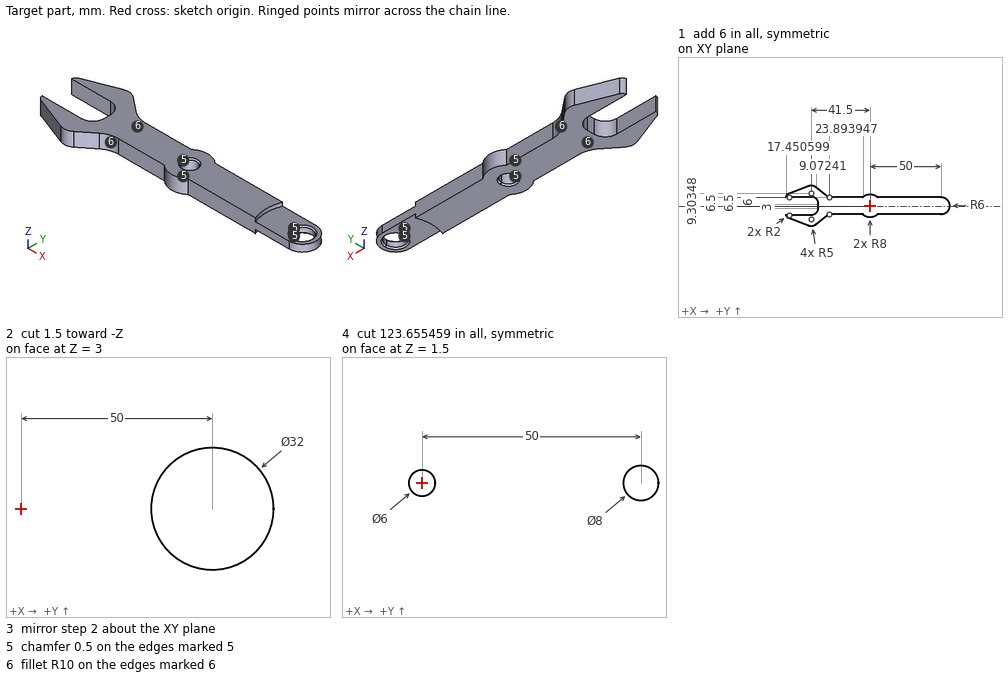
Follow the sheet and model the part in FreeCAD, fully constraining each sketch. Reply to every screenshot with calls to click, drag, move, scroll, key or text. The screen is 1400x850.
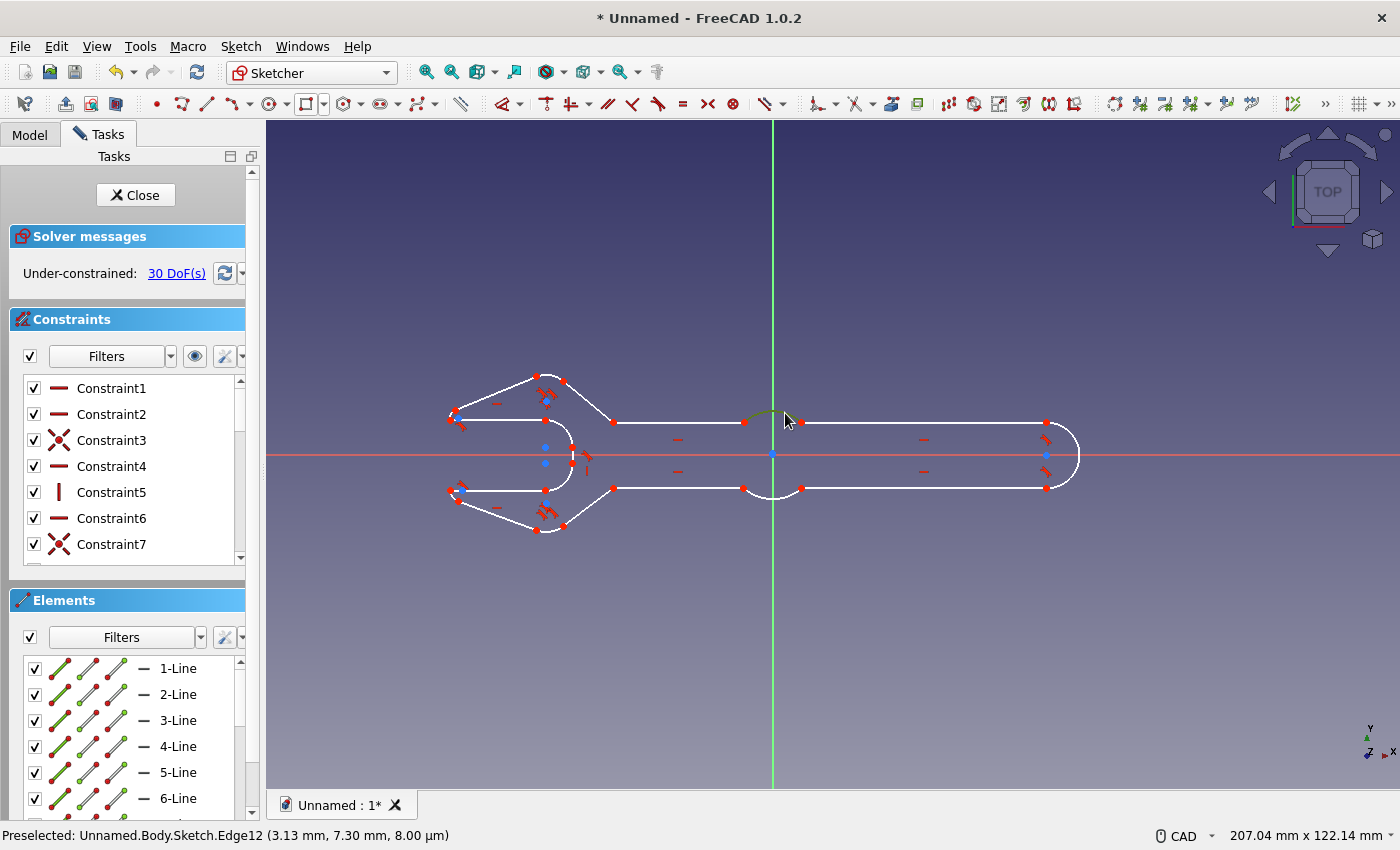
click(760, 497)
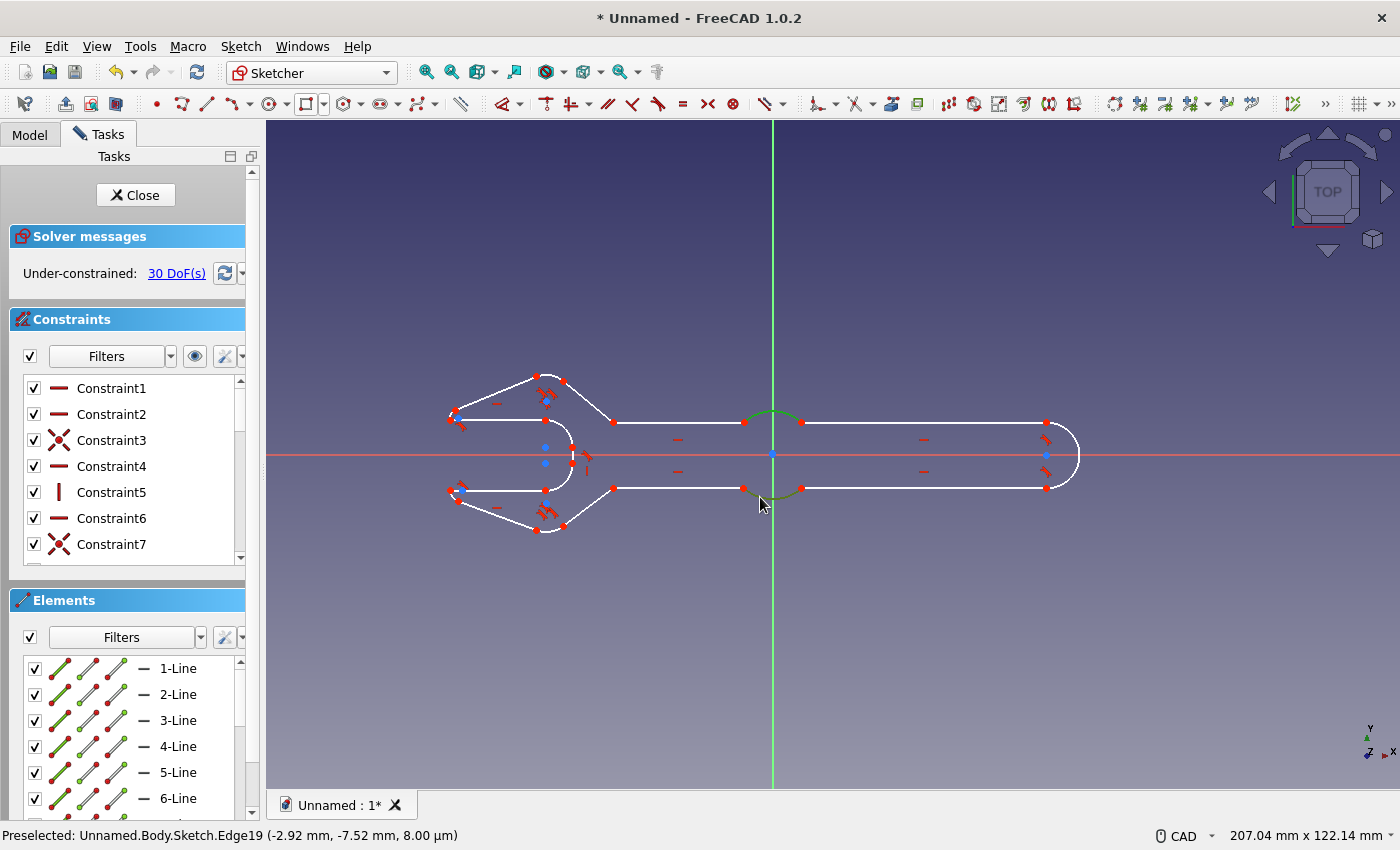
click(546, 104)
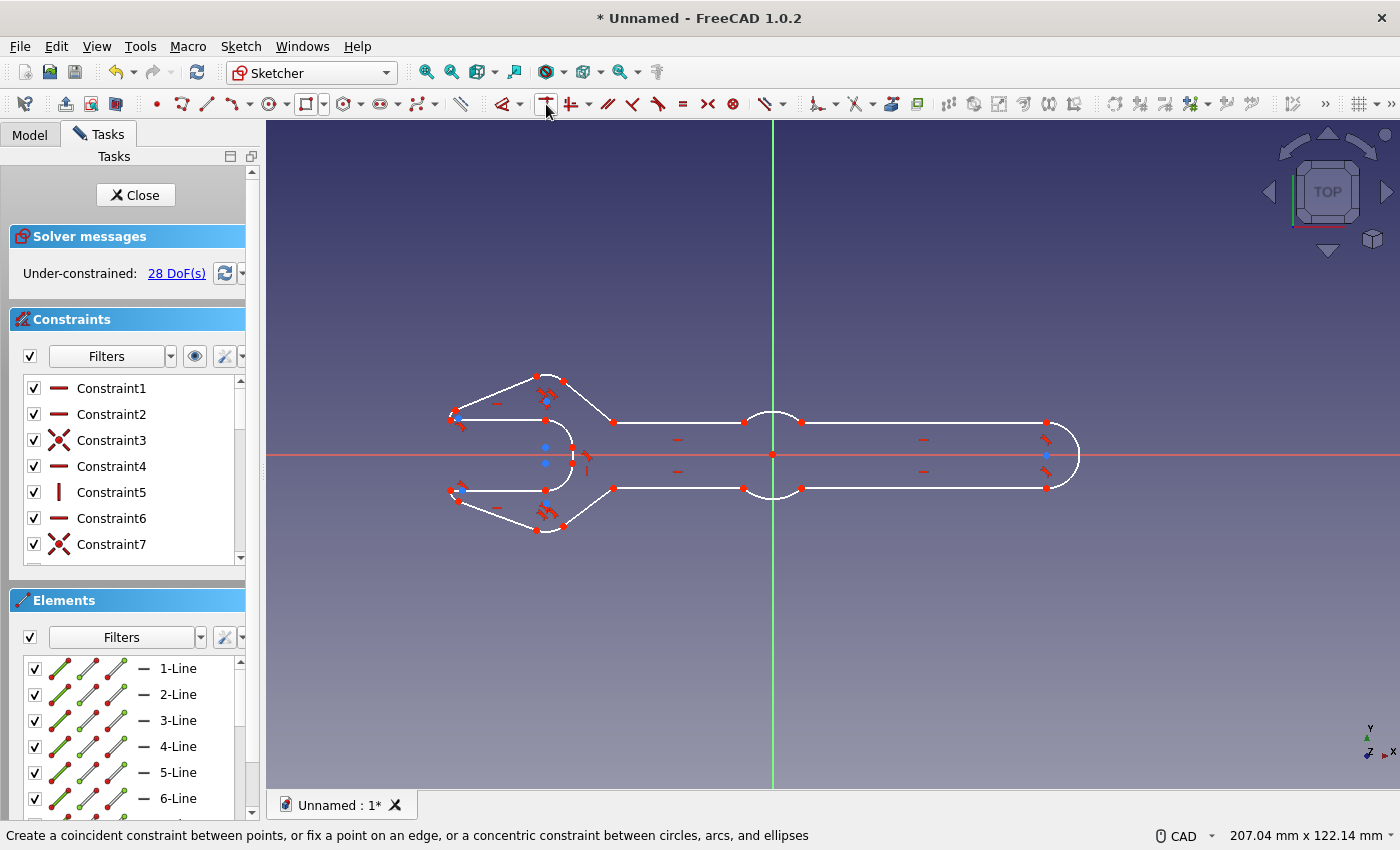
scroll(773, 455, up, 8)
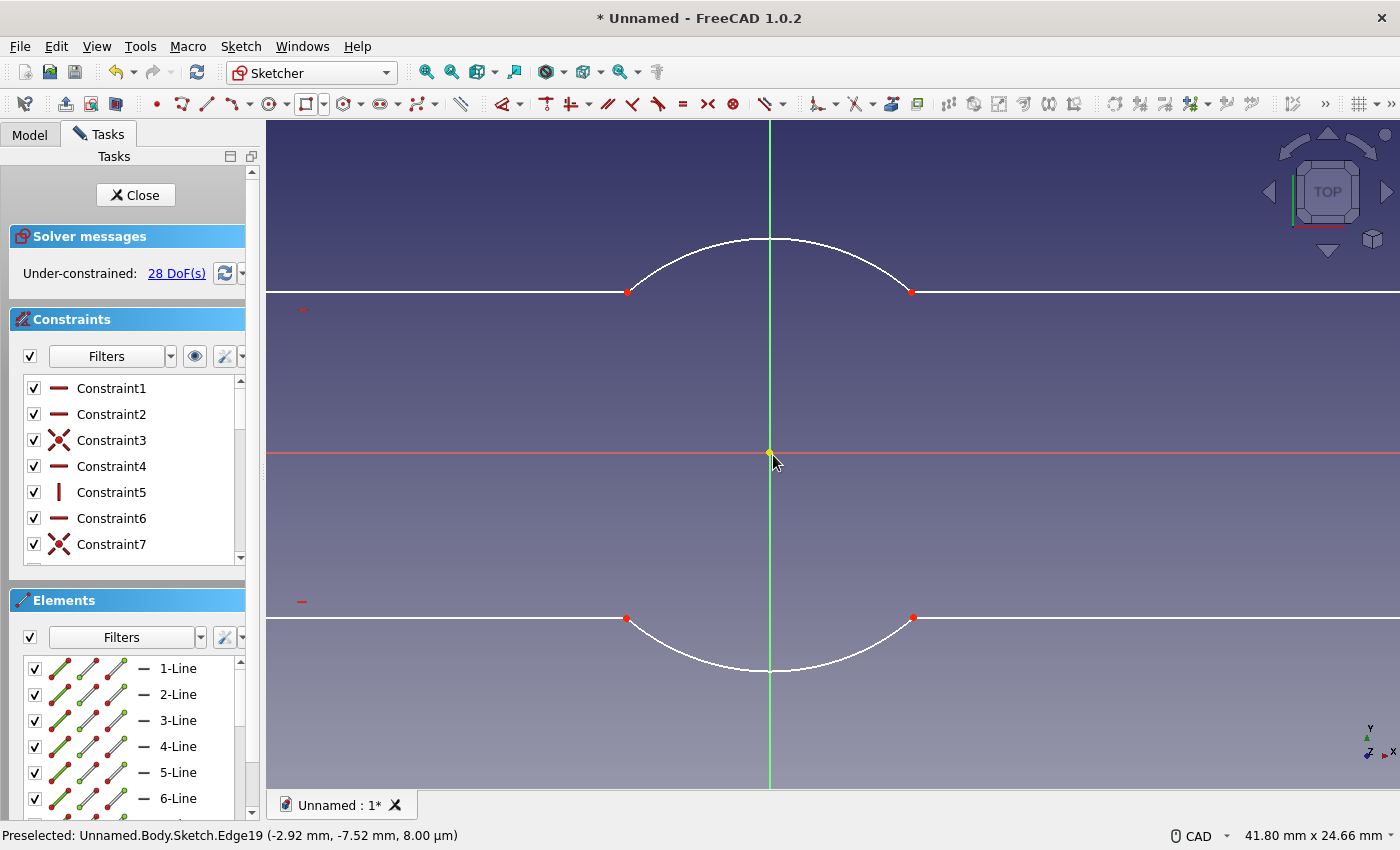
drag(760, 442, 780, 463)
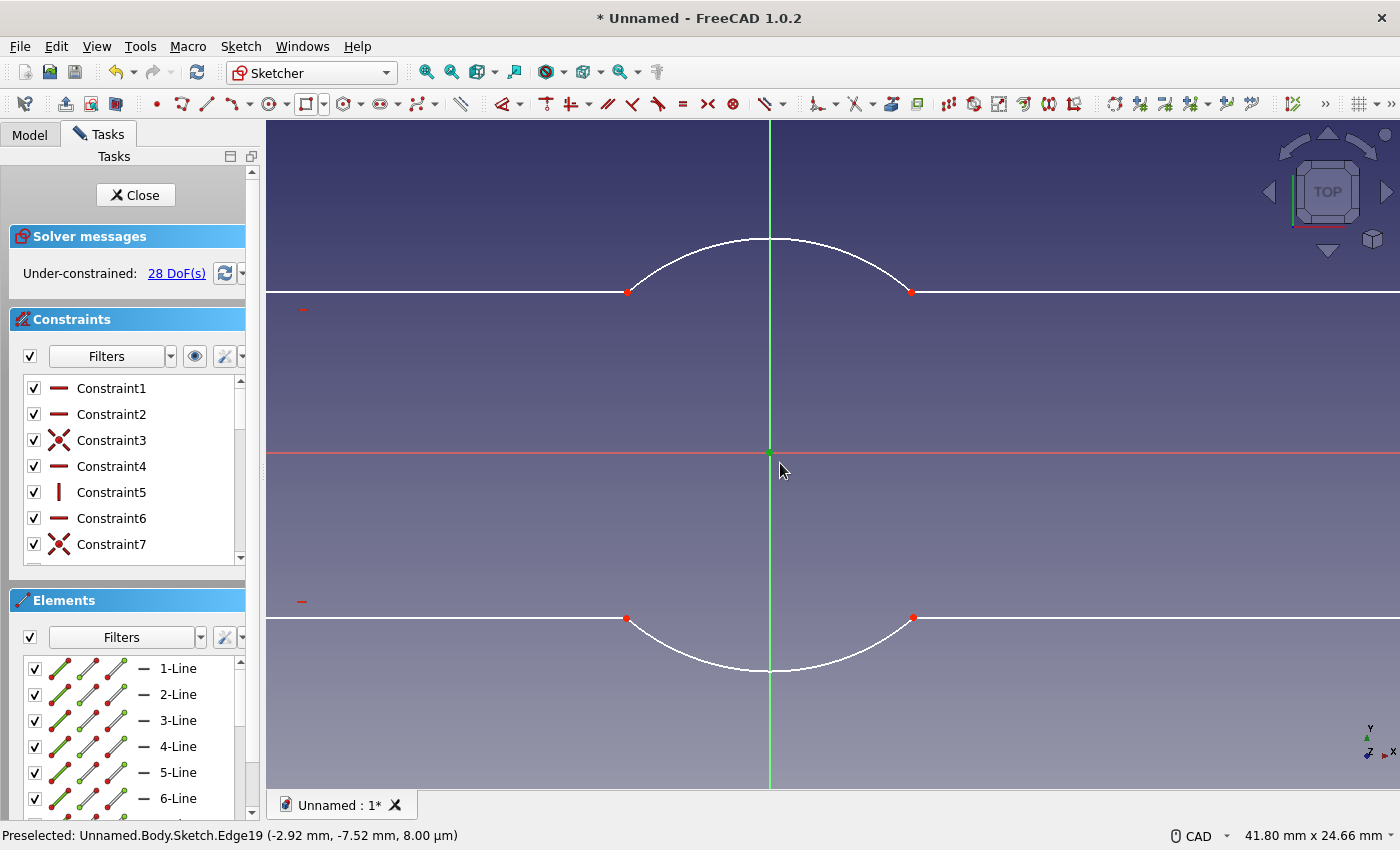
click(546, 104)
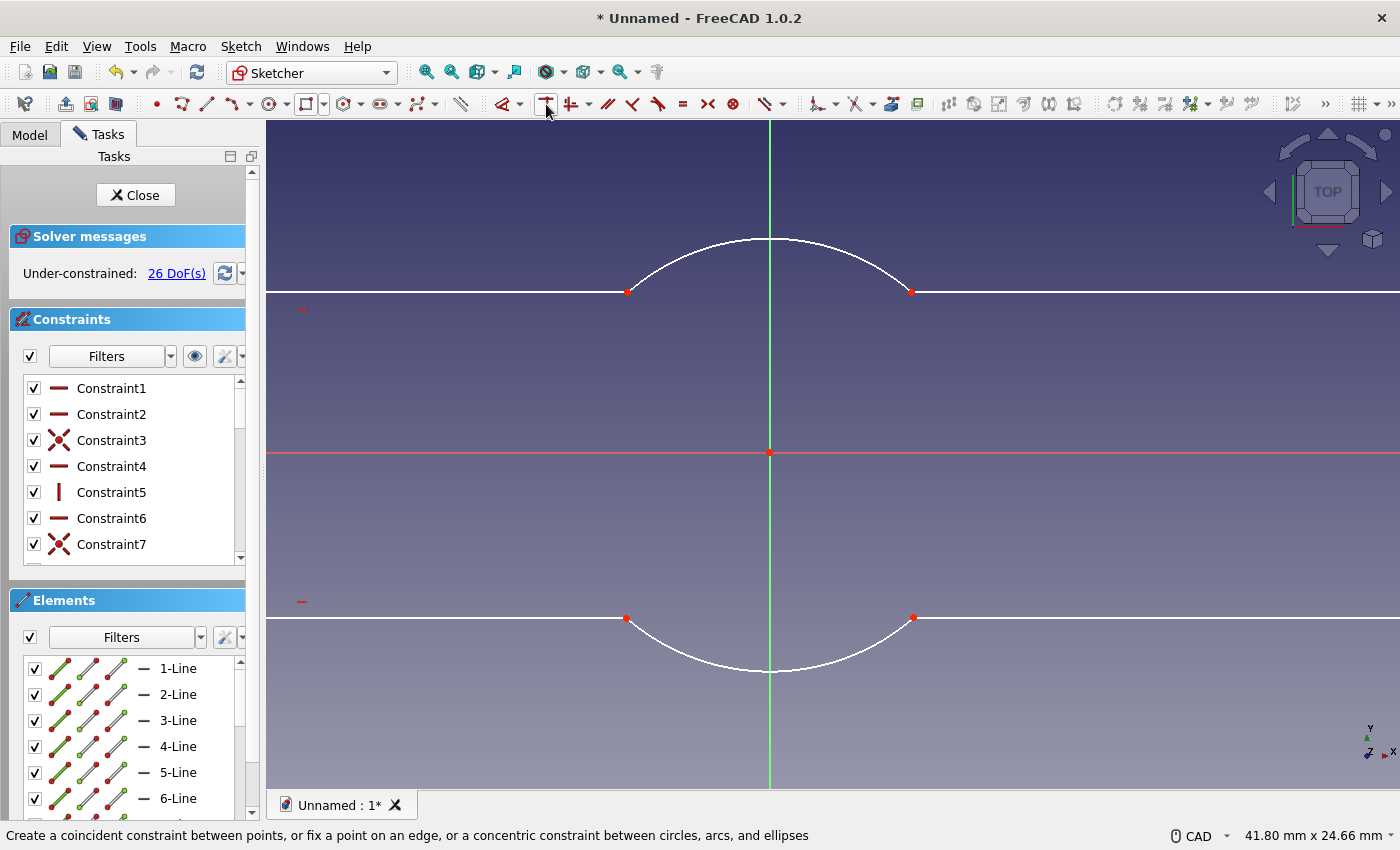
scroll(773, 455, down, 8)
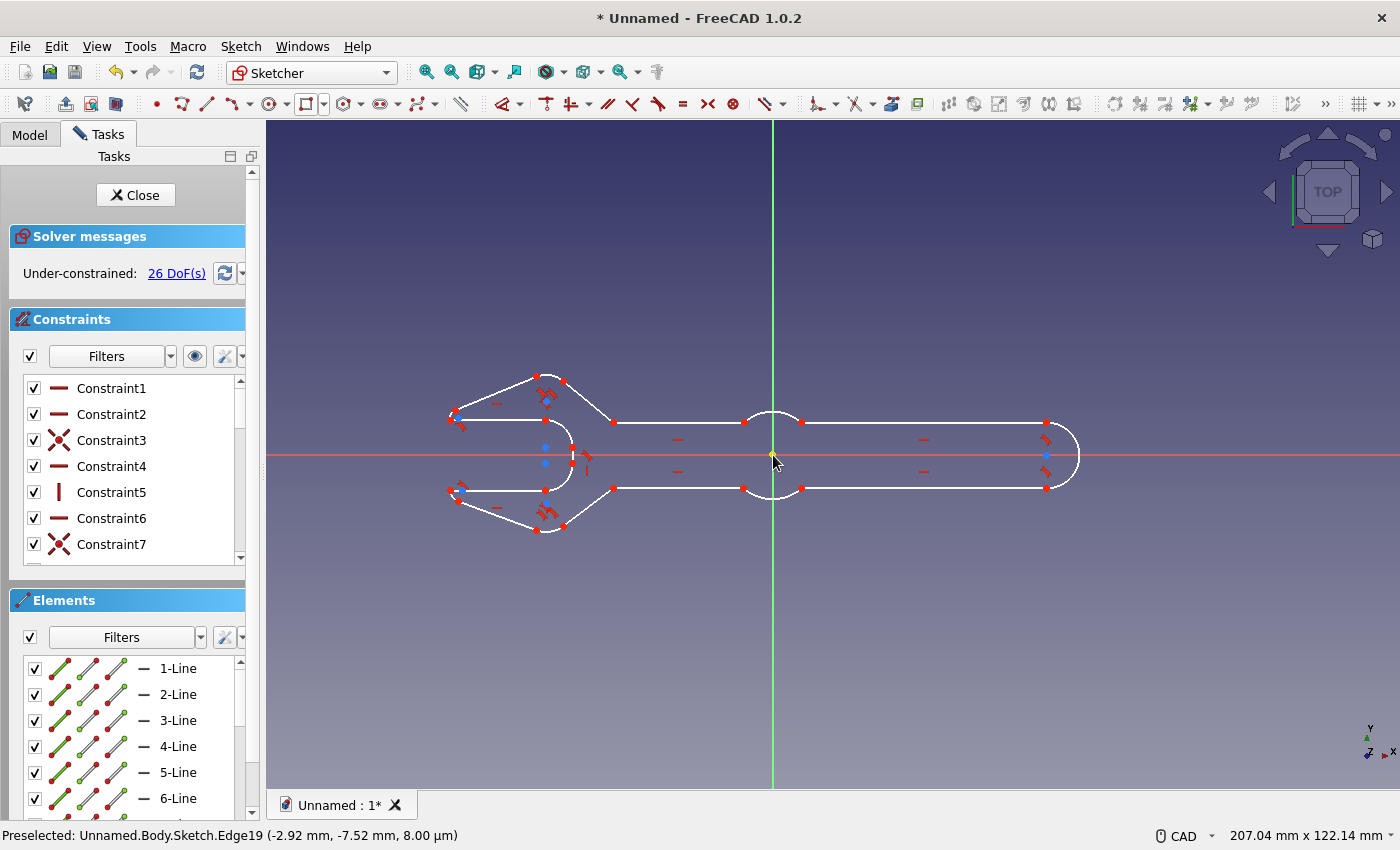
scroll(556, 377, up, 3)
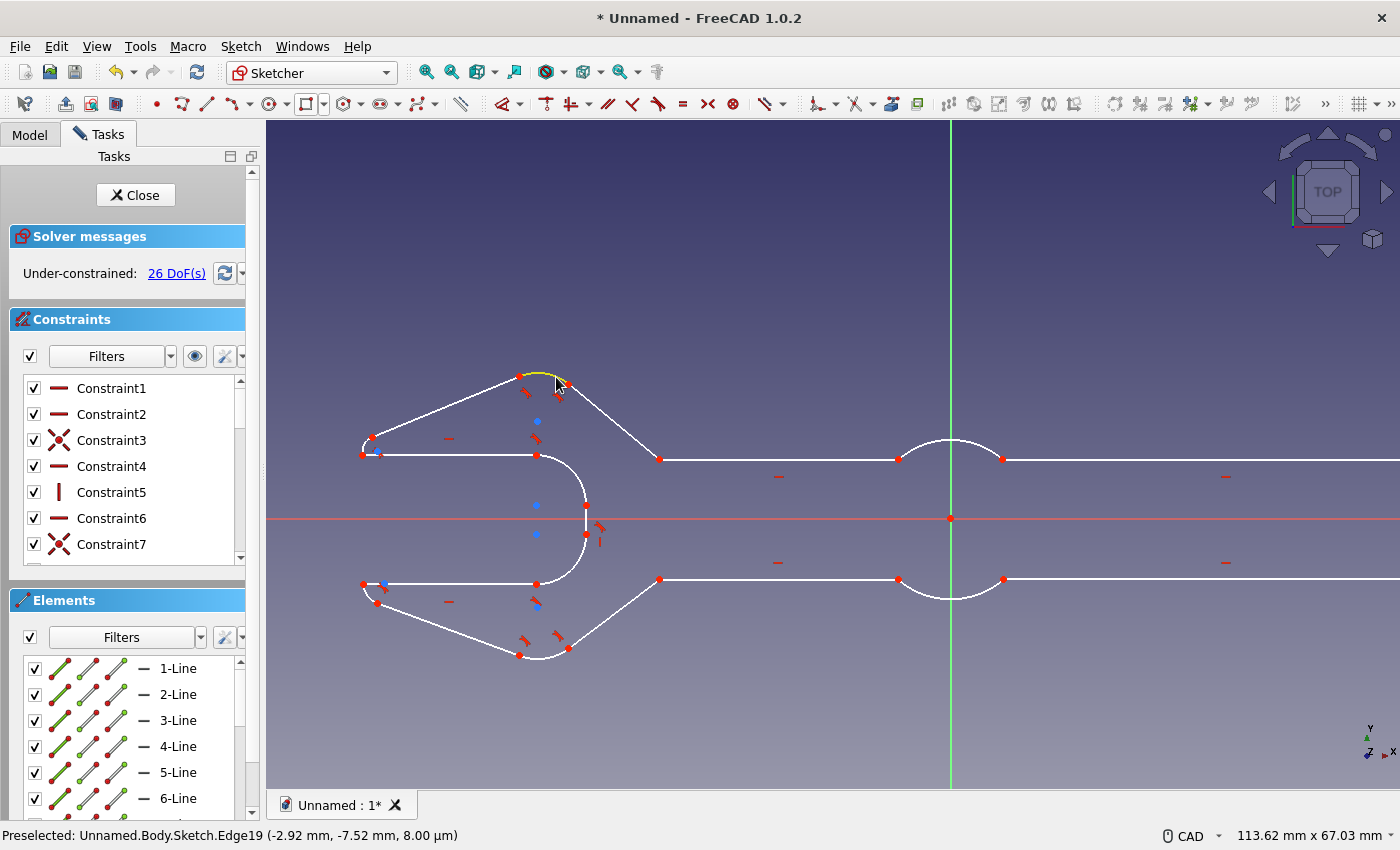
click(555, 376)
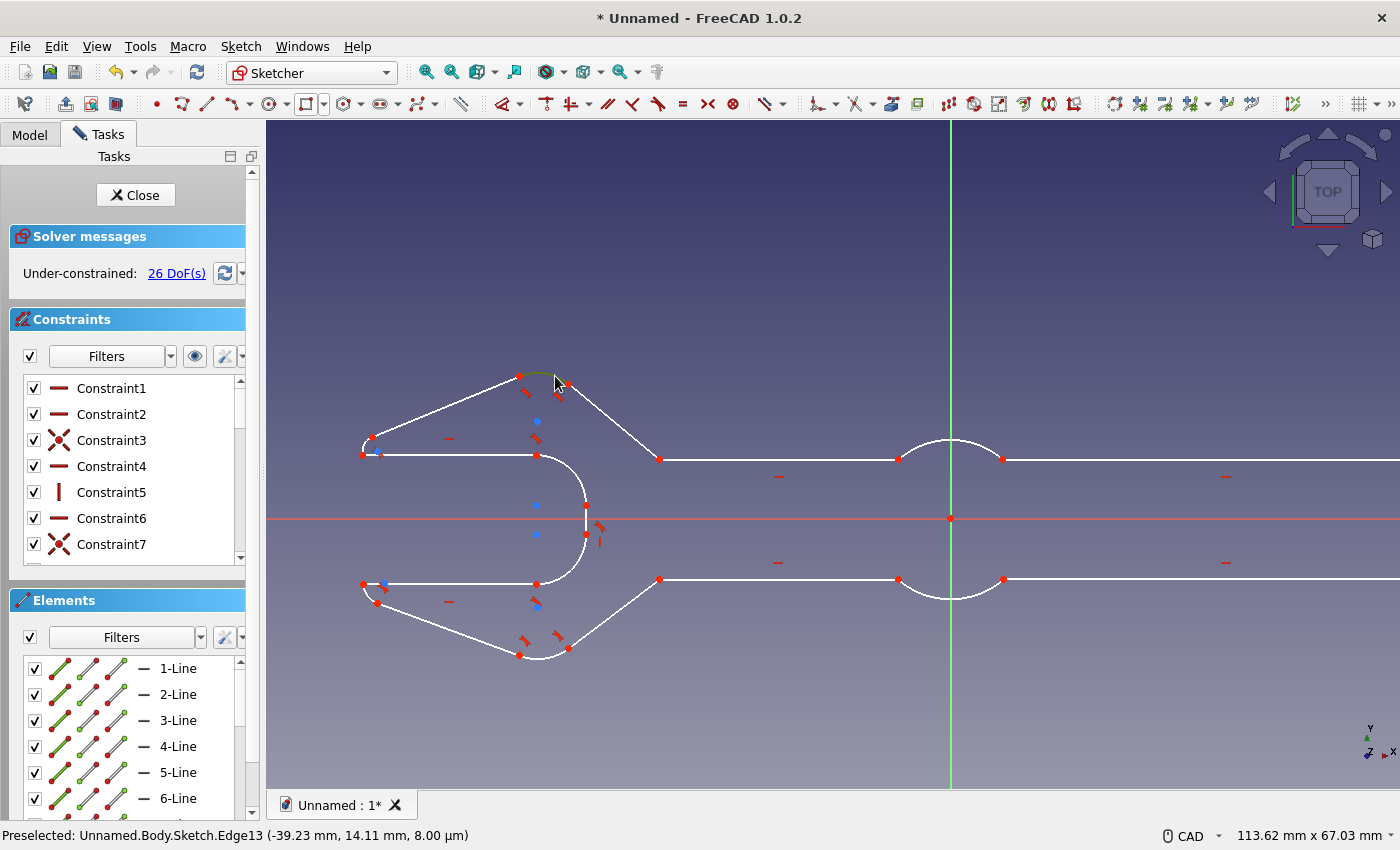
click(581, 483)